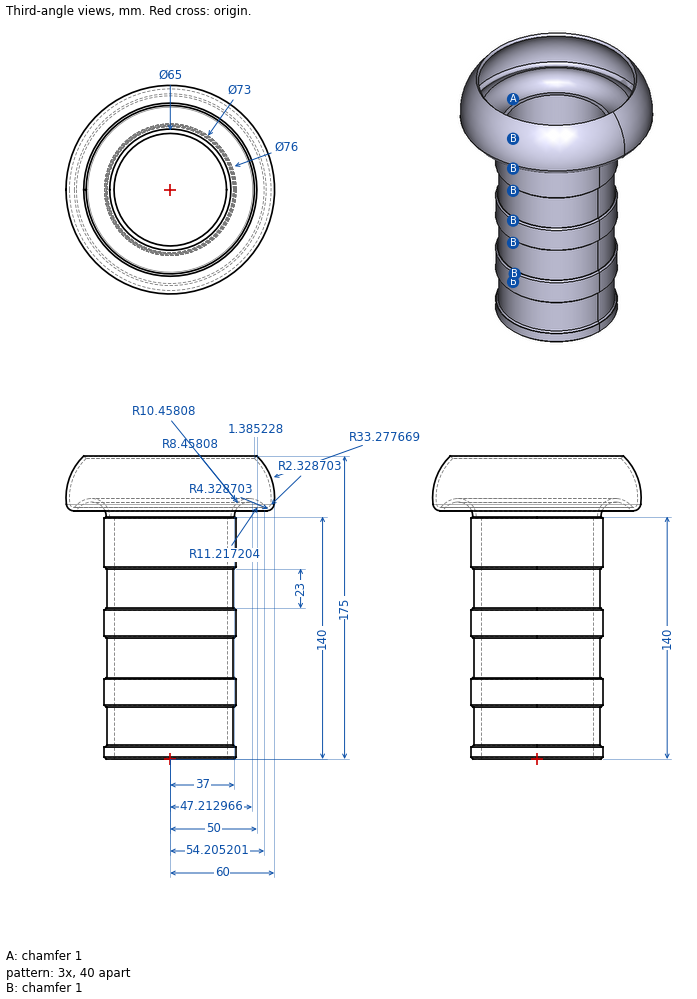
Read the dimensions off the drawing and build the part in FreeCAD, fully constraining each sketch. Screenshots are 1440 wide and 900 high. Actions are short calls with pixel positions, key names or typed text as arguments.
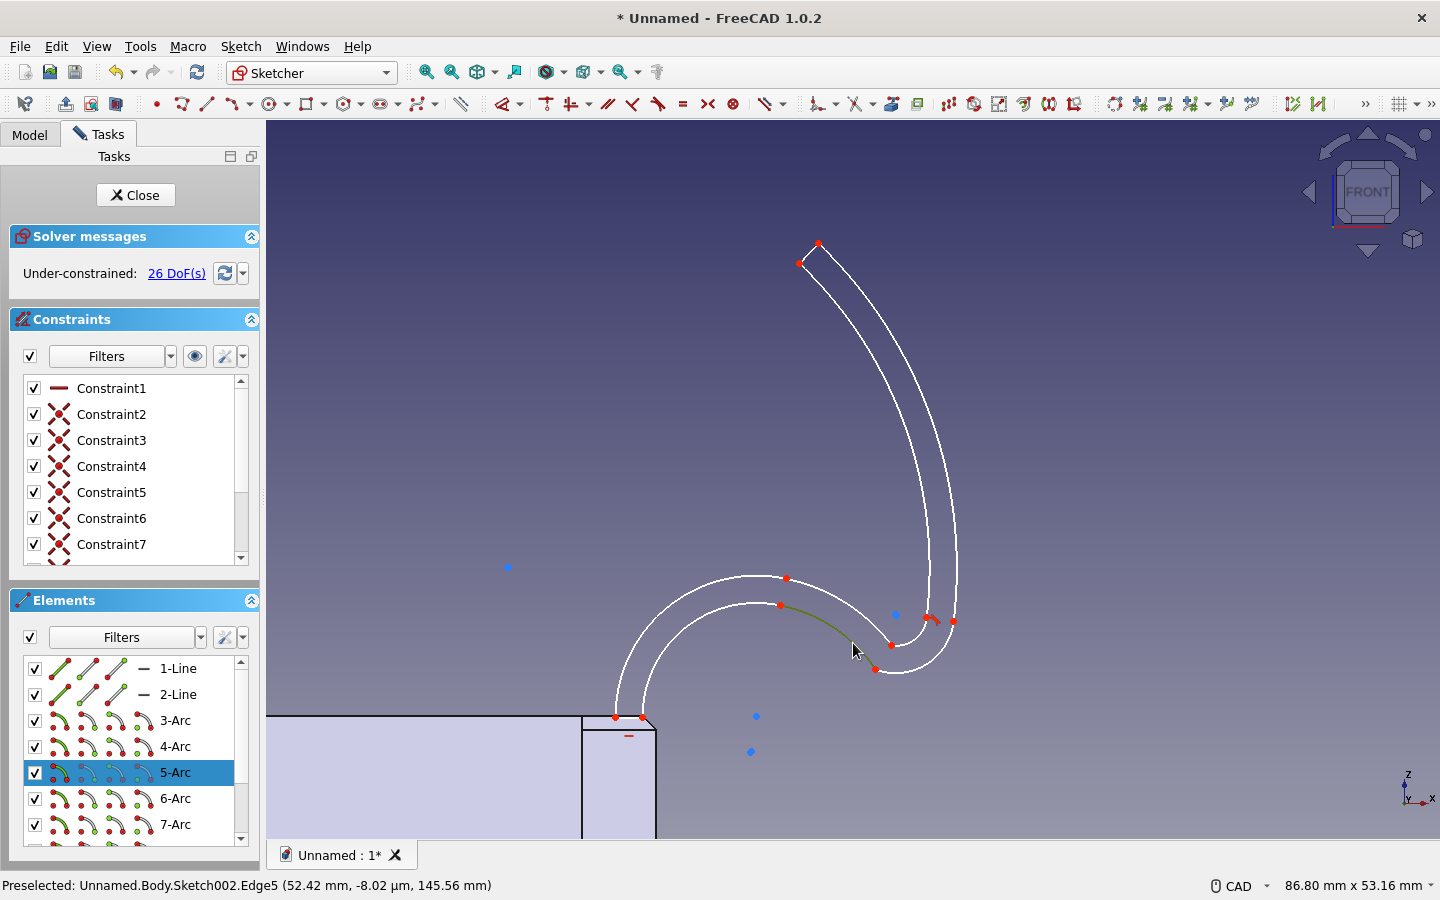
click(720, 609)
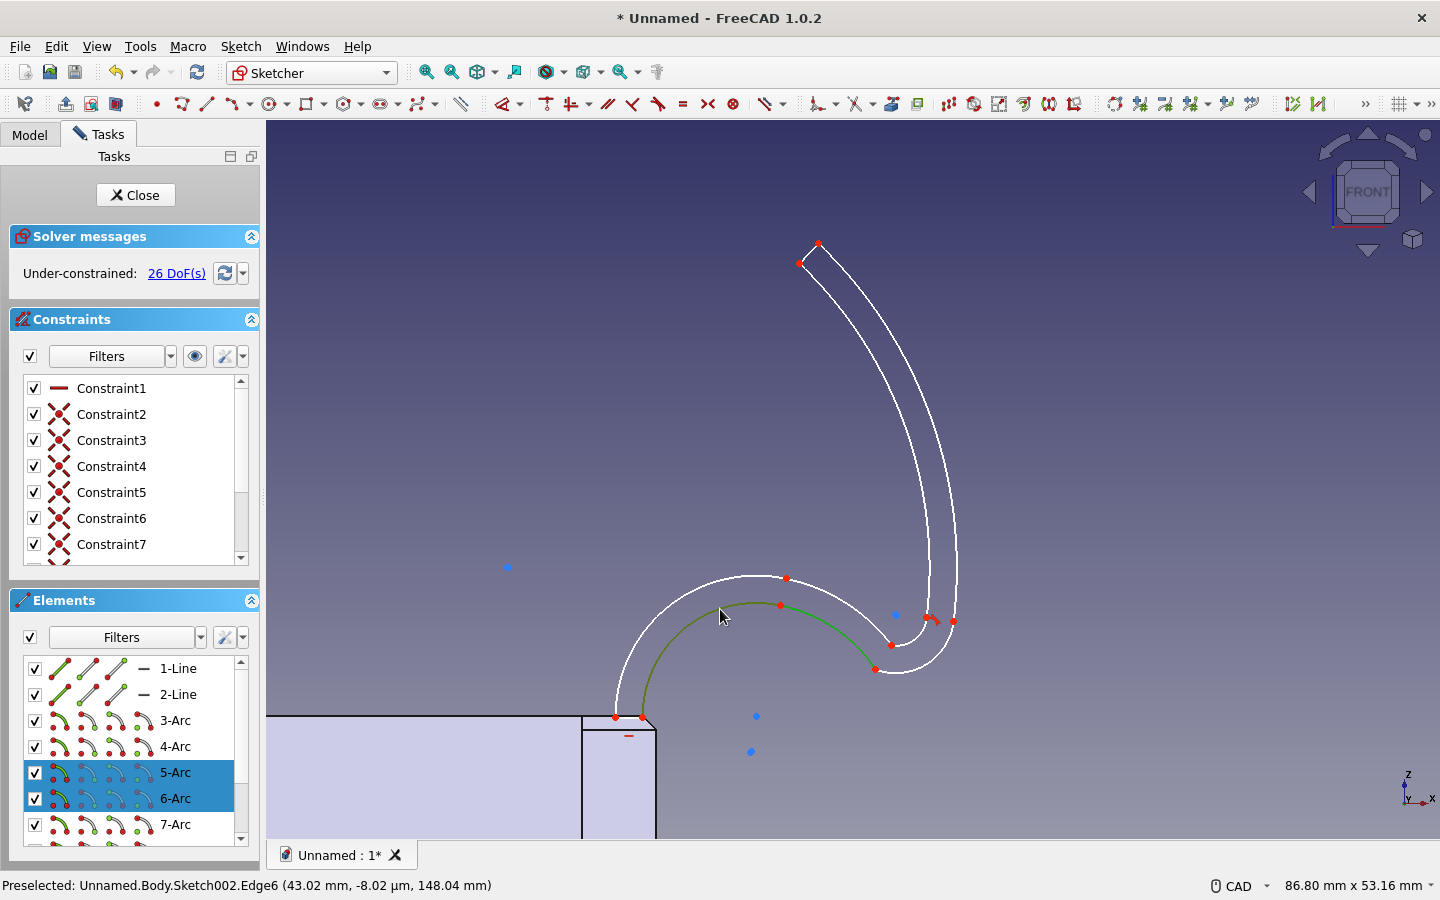
click(658, 104)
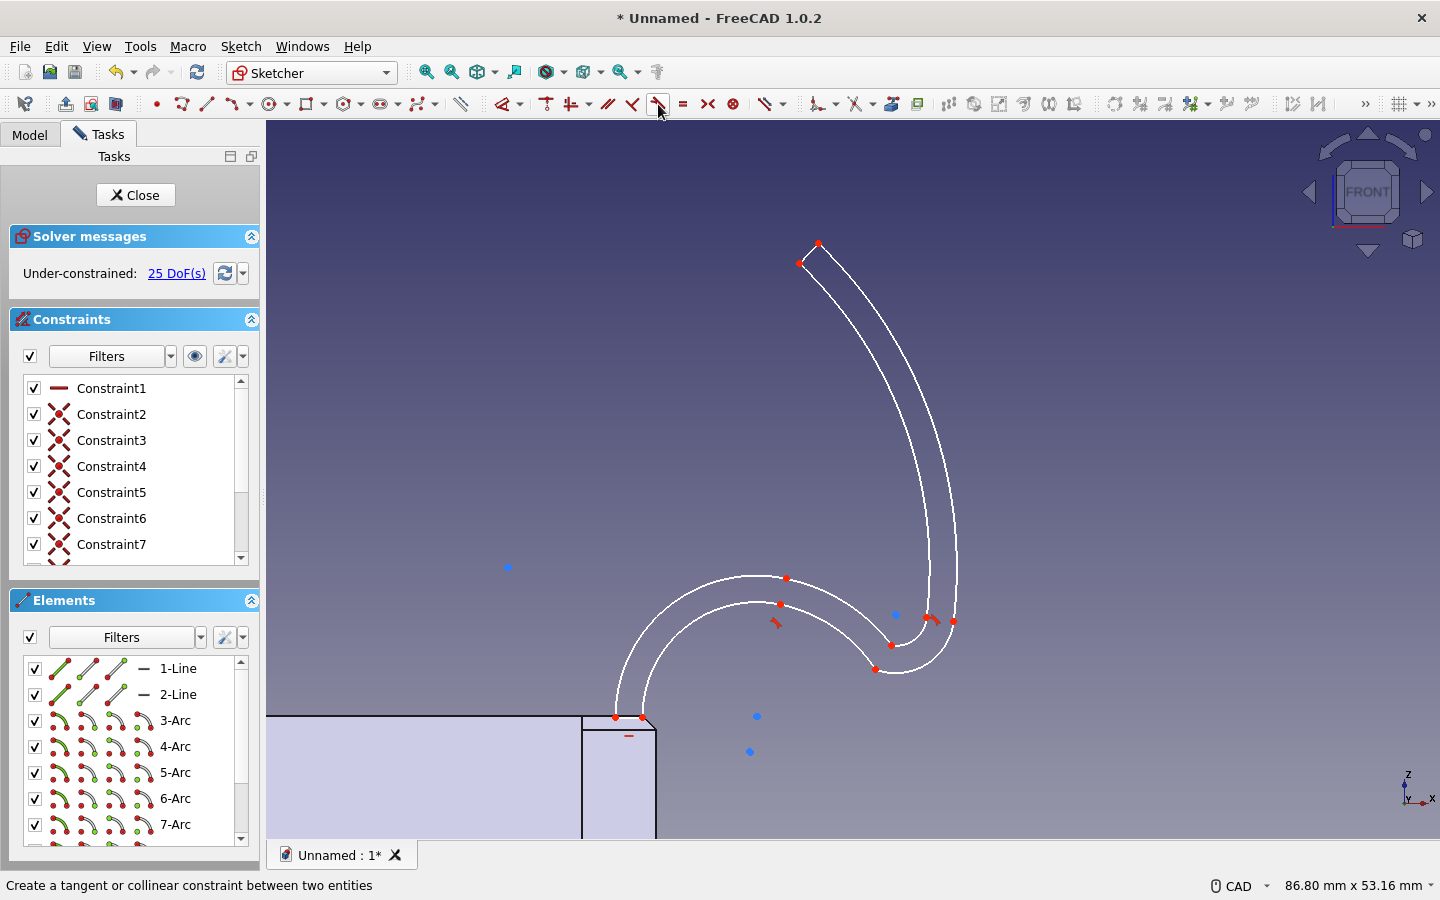
click(712, 583)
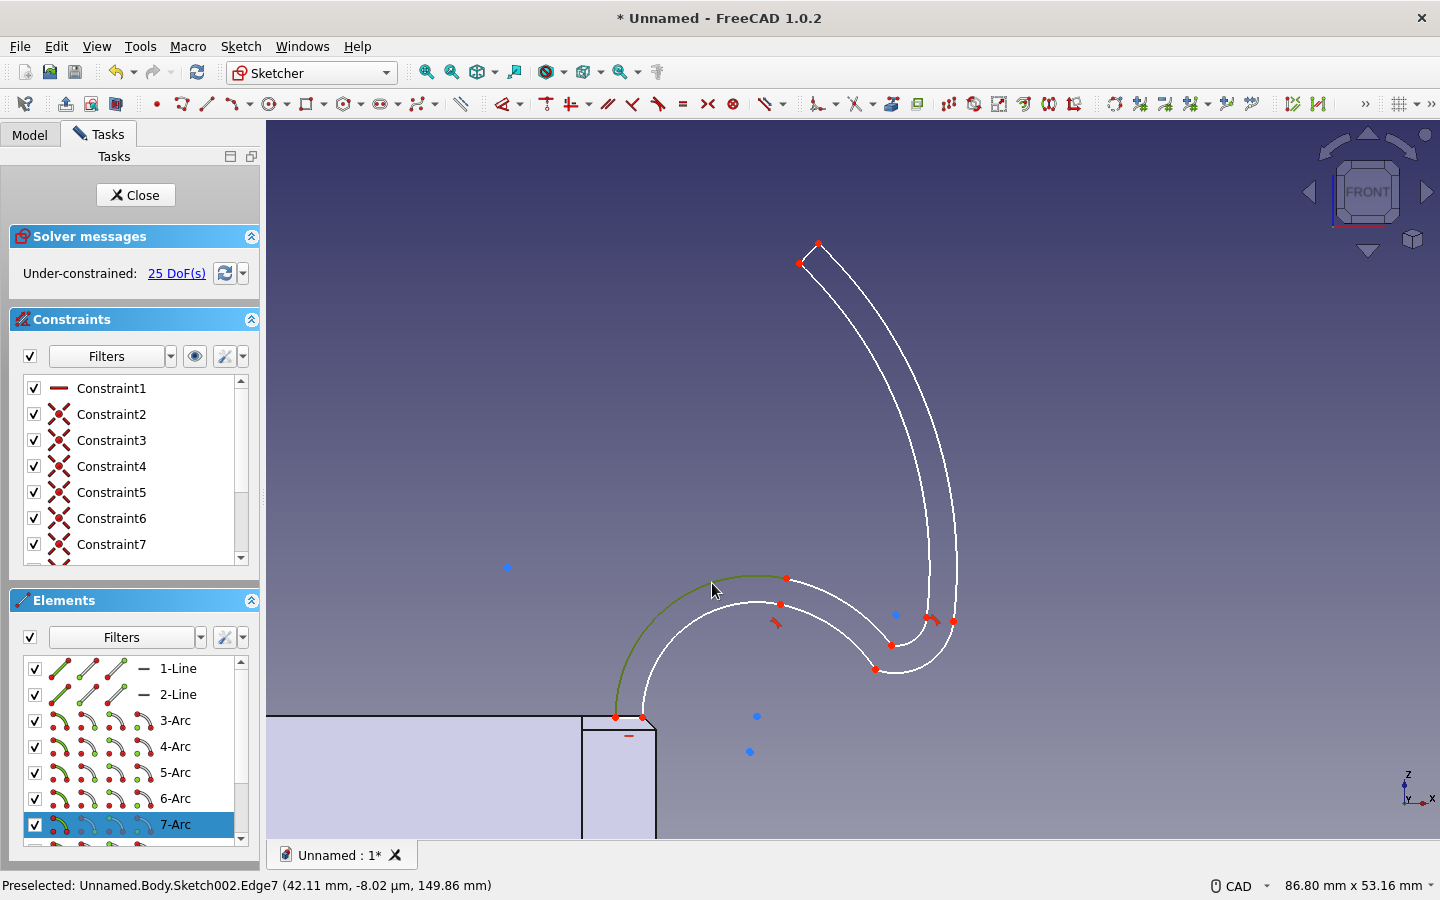
click(866, 618)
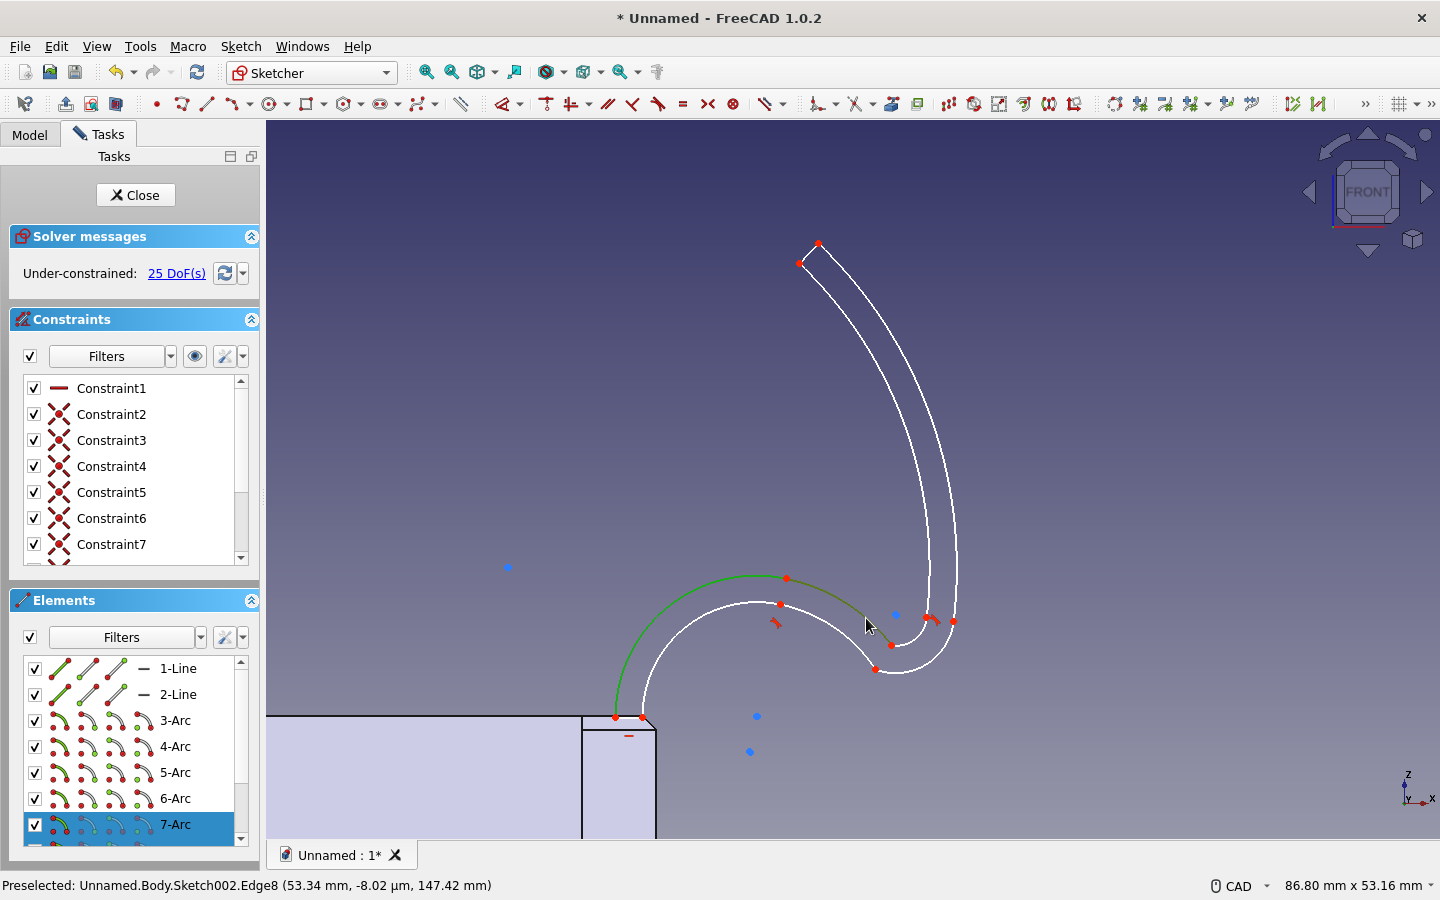
key(t)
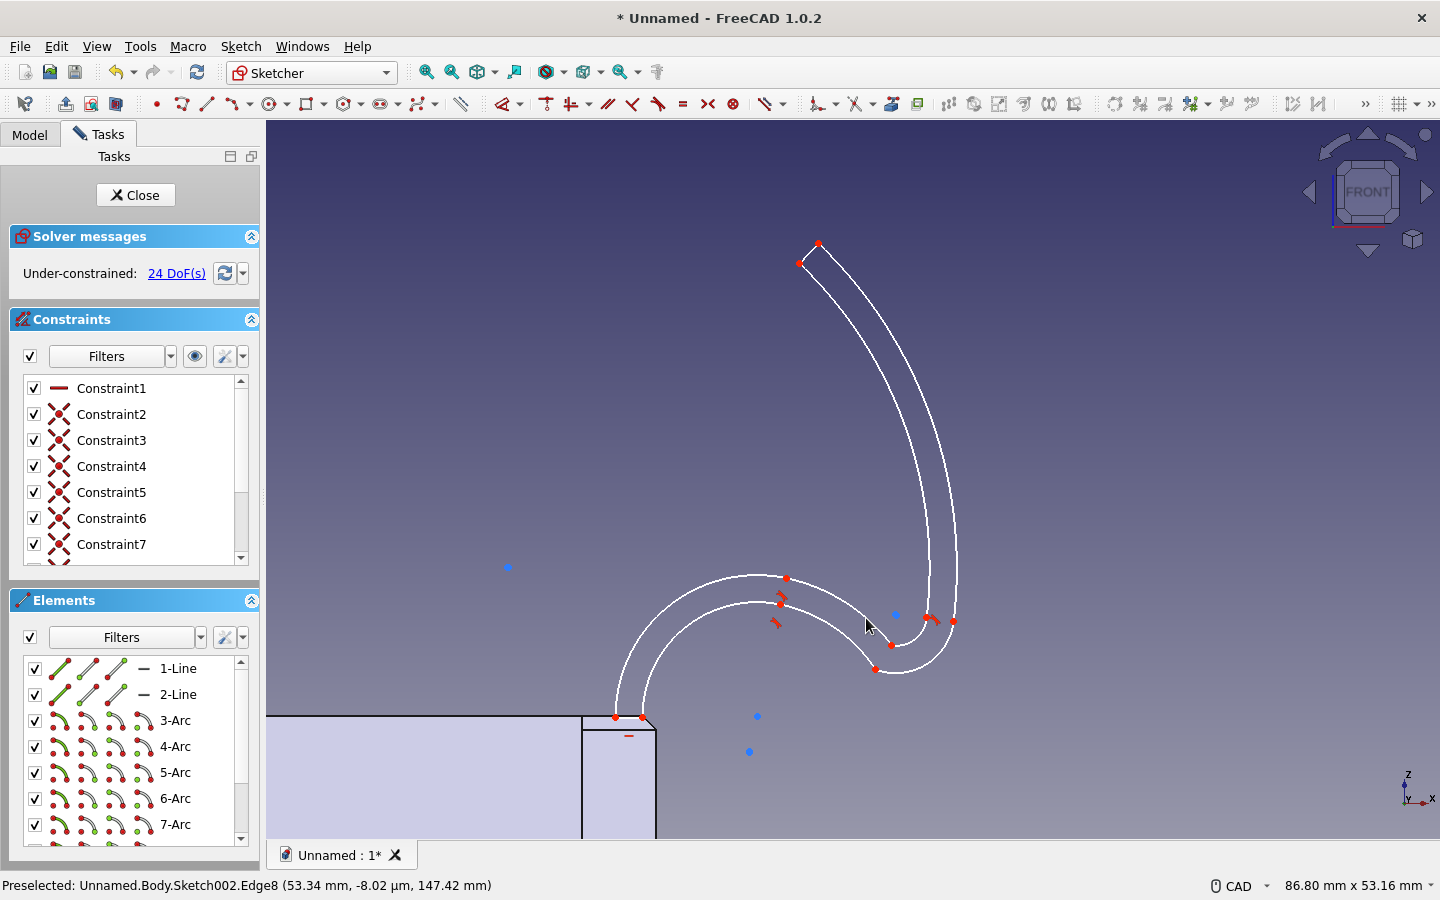
click(907, 644)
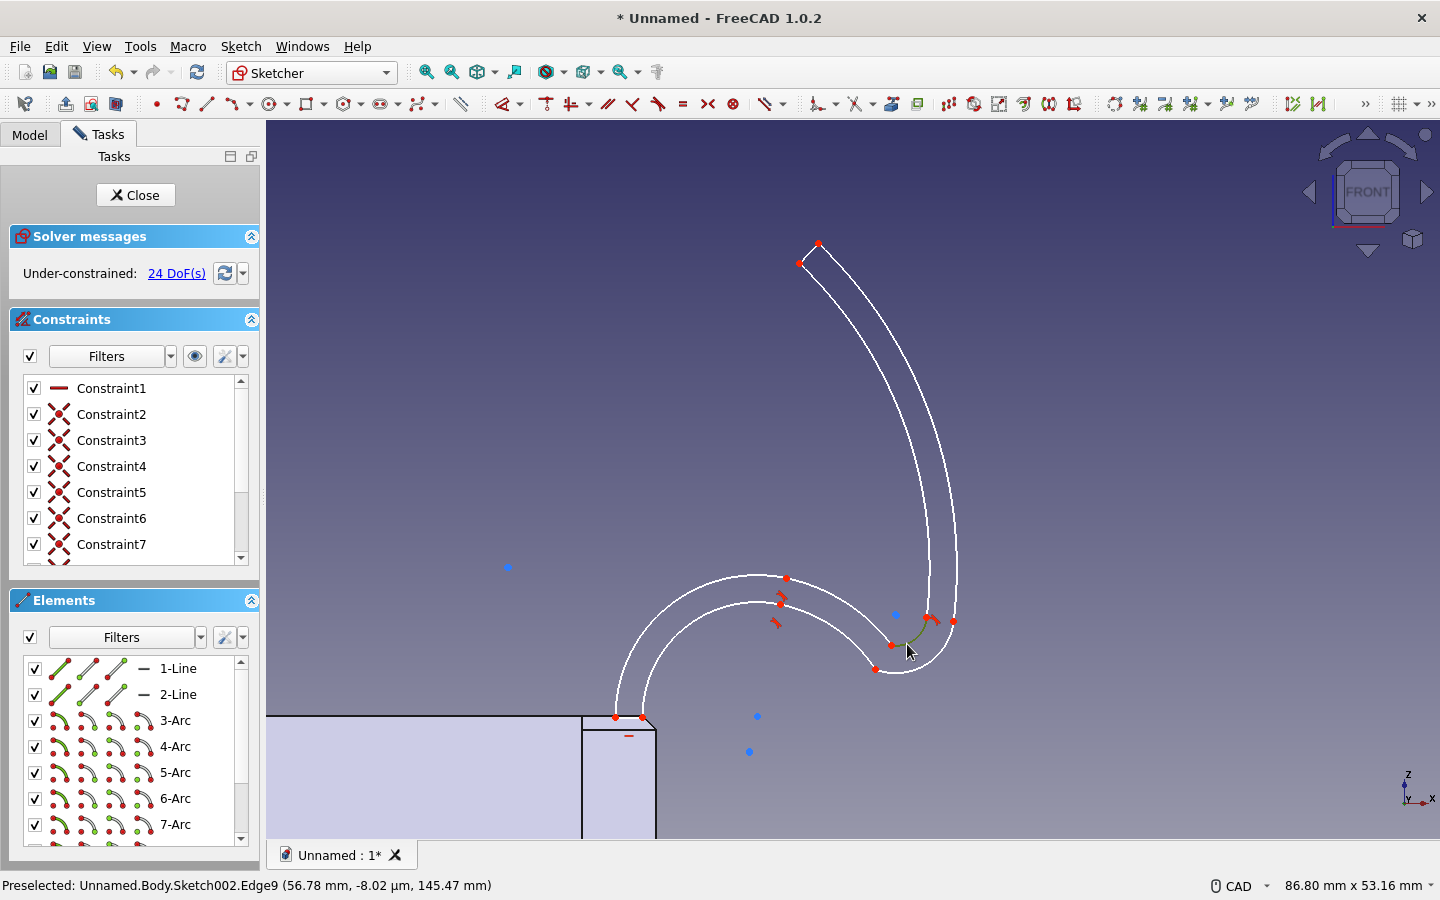
click(924, 501)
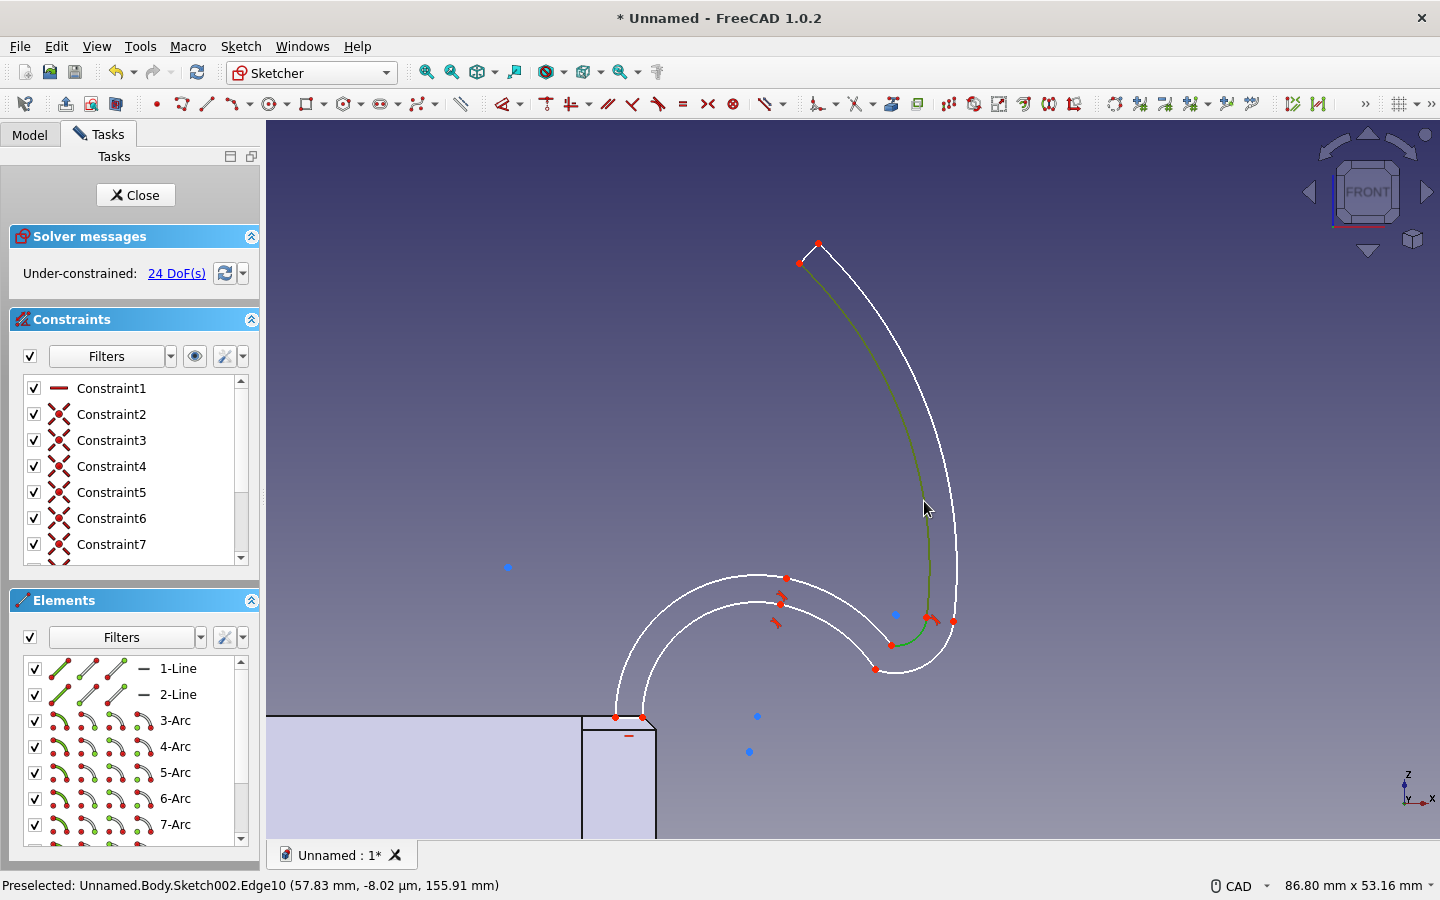
key(t)